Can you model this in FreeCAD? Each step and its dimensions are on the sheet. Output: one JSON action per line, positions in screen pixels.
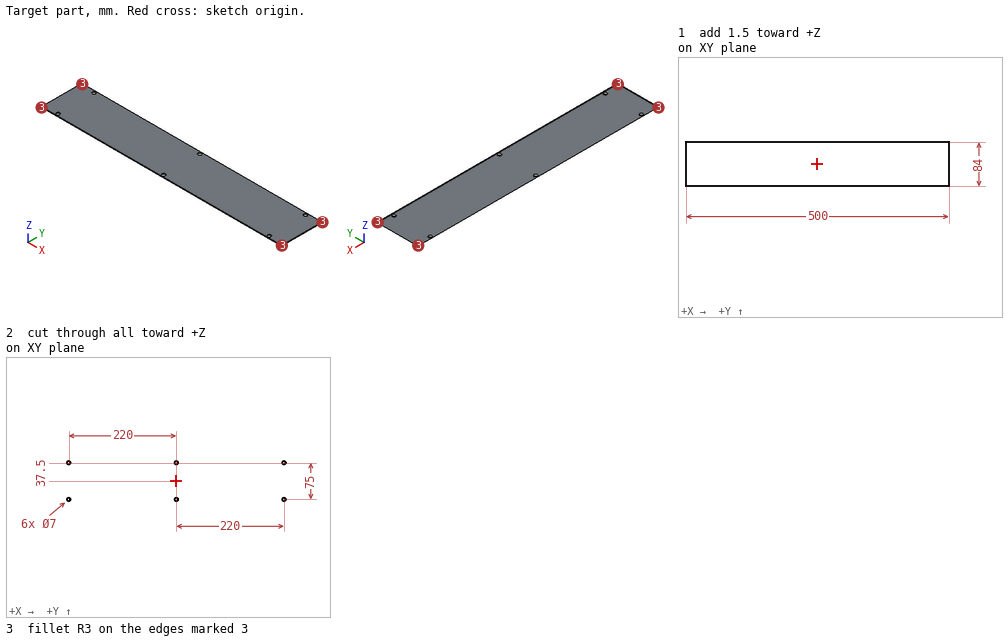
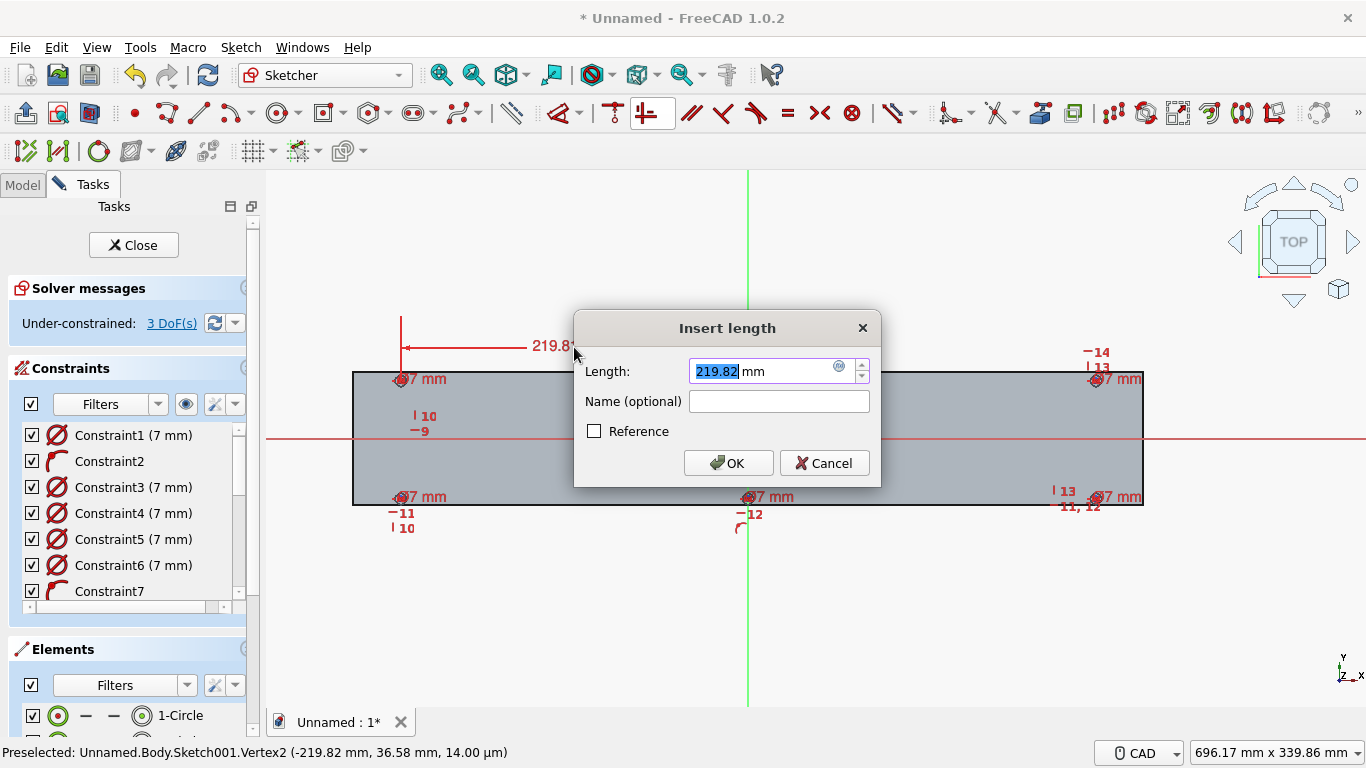
{"action": "type", "text": "220"}
{"action": "key", "text": "Return"}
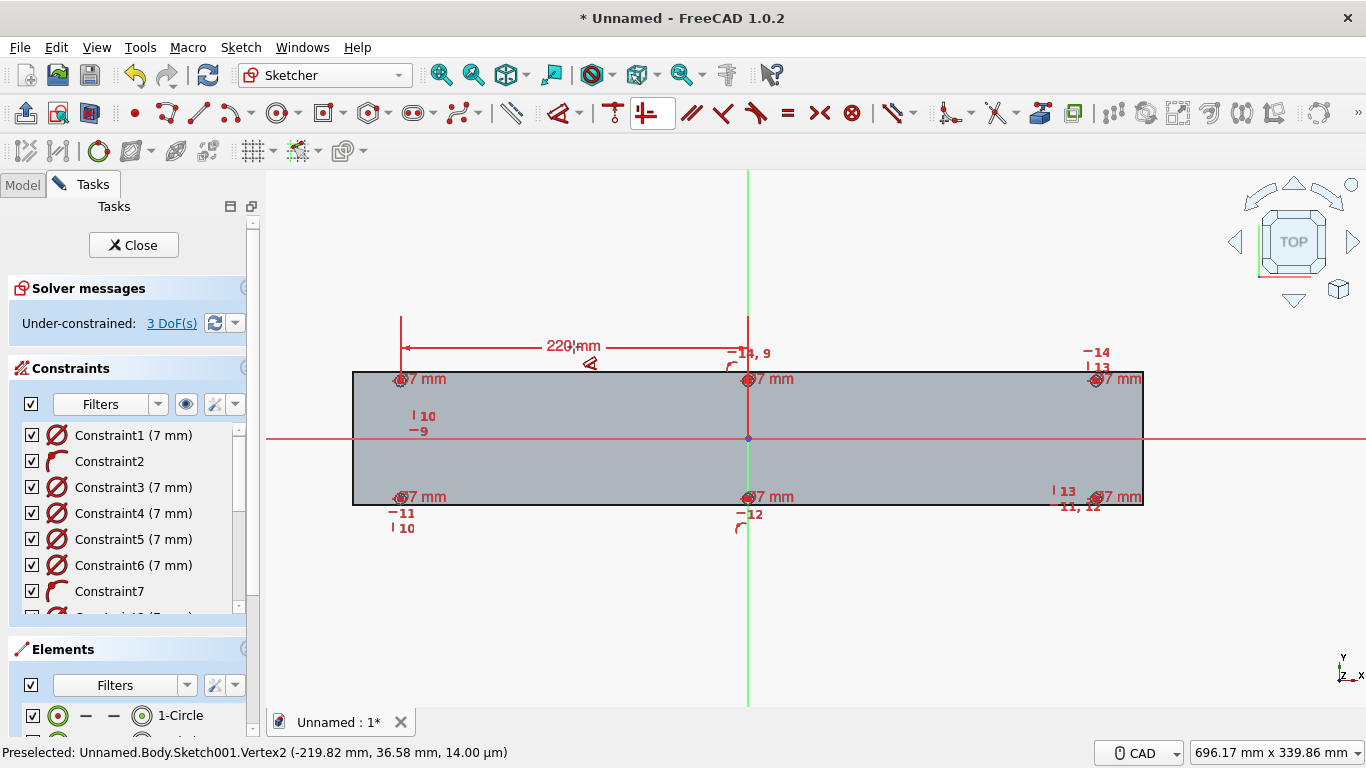
{"action": "left_click", "coordinate": [1096, 499]}
{"action": "left_click", "coordinate": [922, 533]}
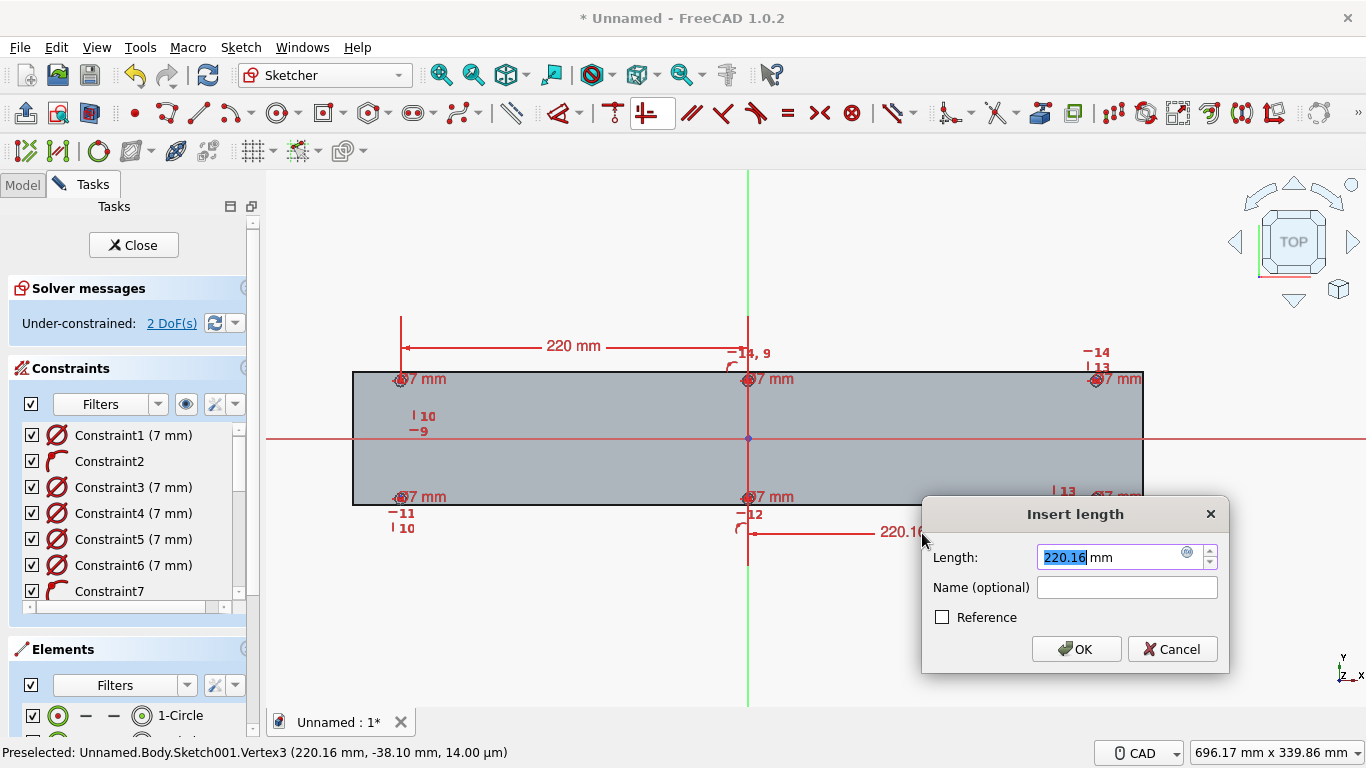
{"action": "type", "text": "220"}
{"action": "key", "text": "Return"}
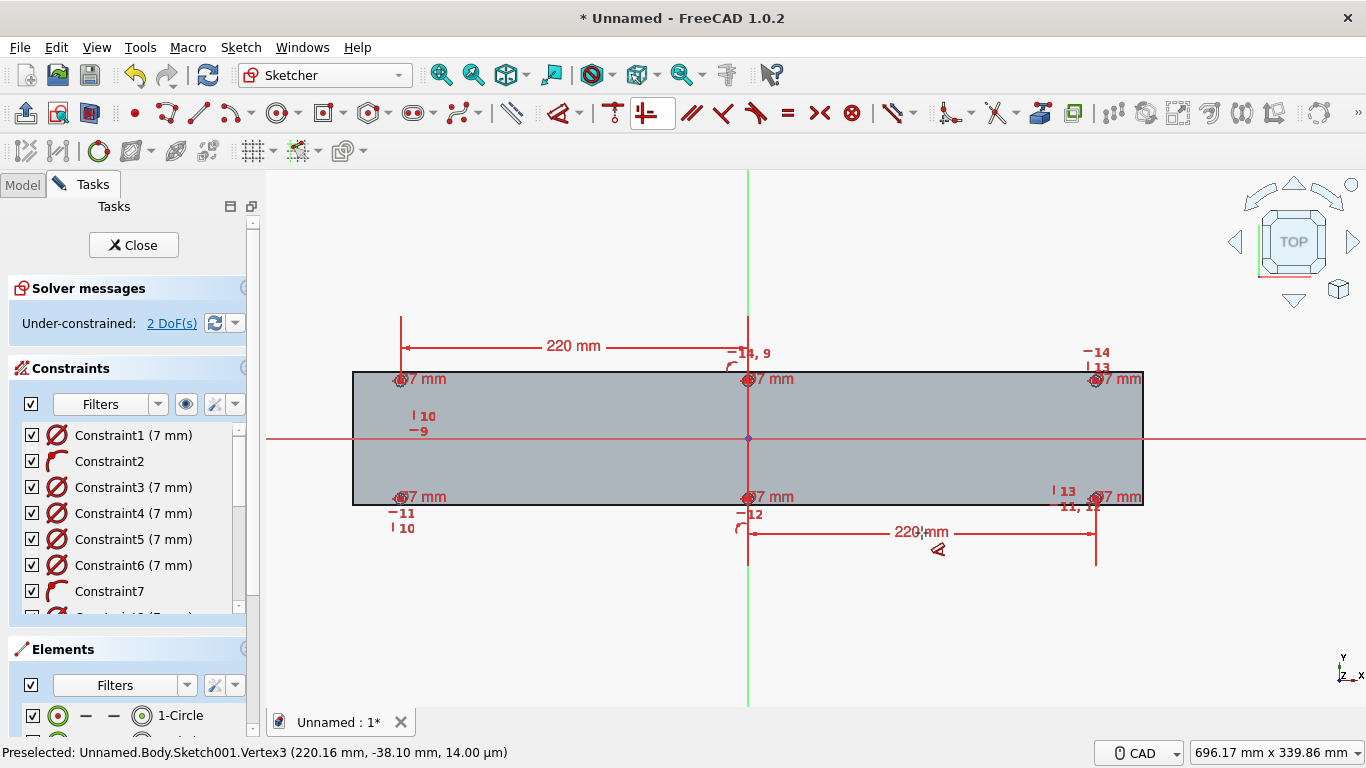
{"action": "left_click", "coordinate": [748, 381]}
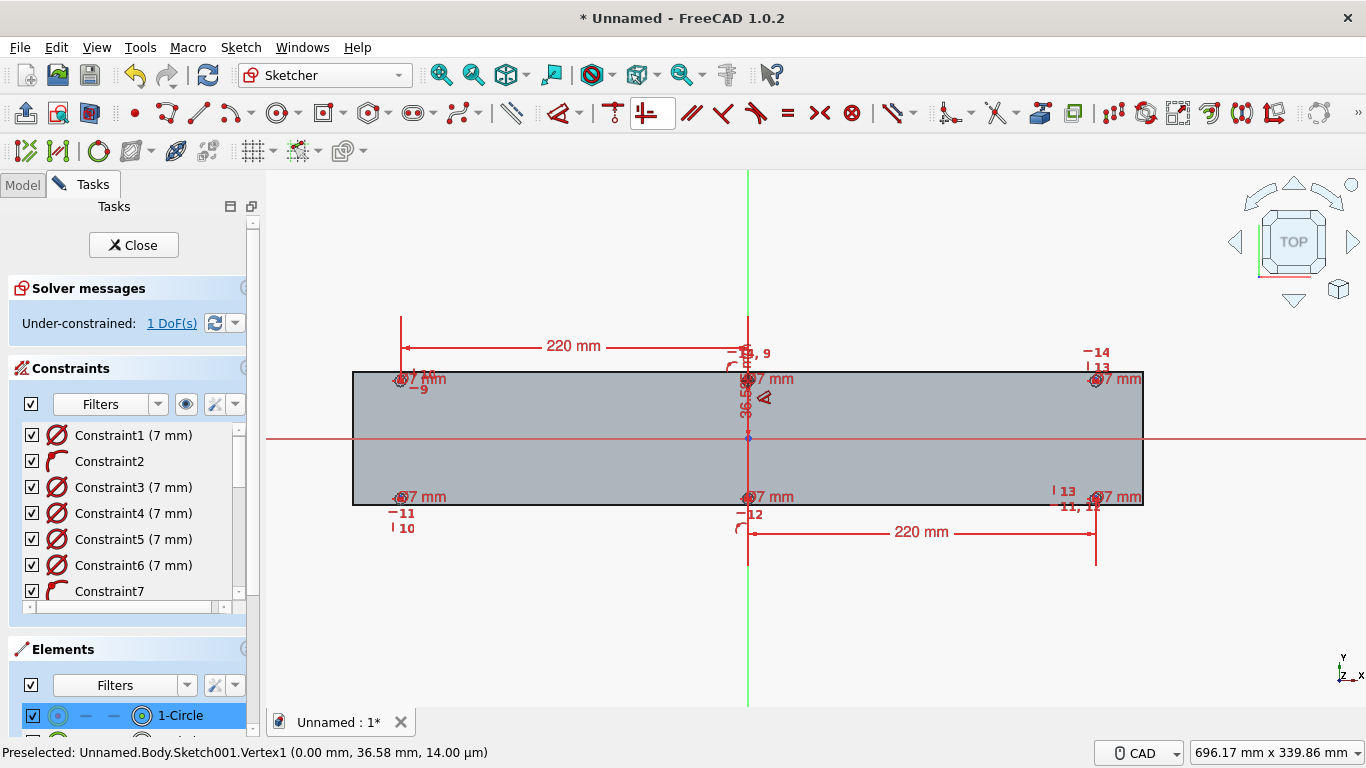
{"action": "left_click", "coordinate": [1096, 499]}
{"action": "left_click", "coordinate": [1130, 413]}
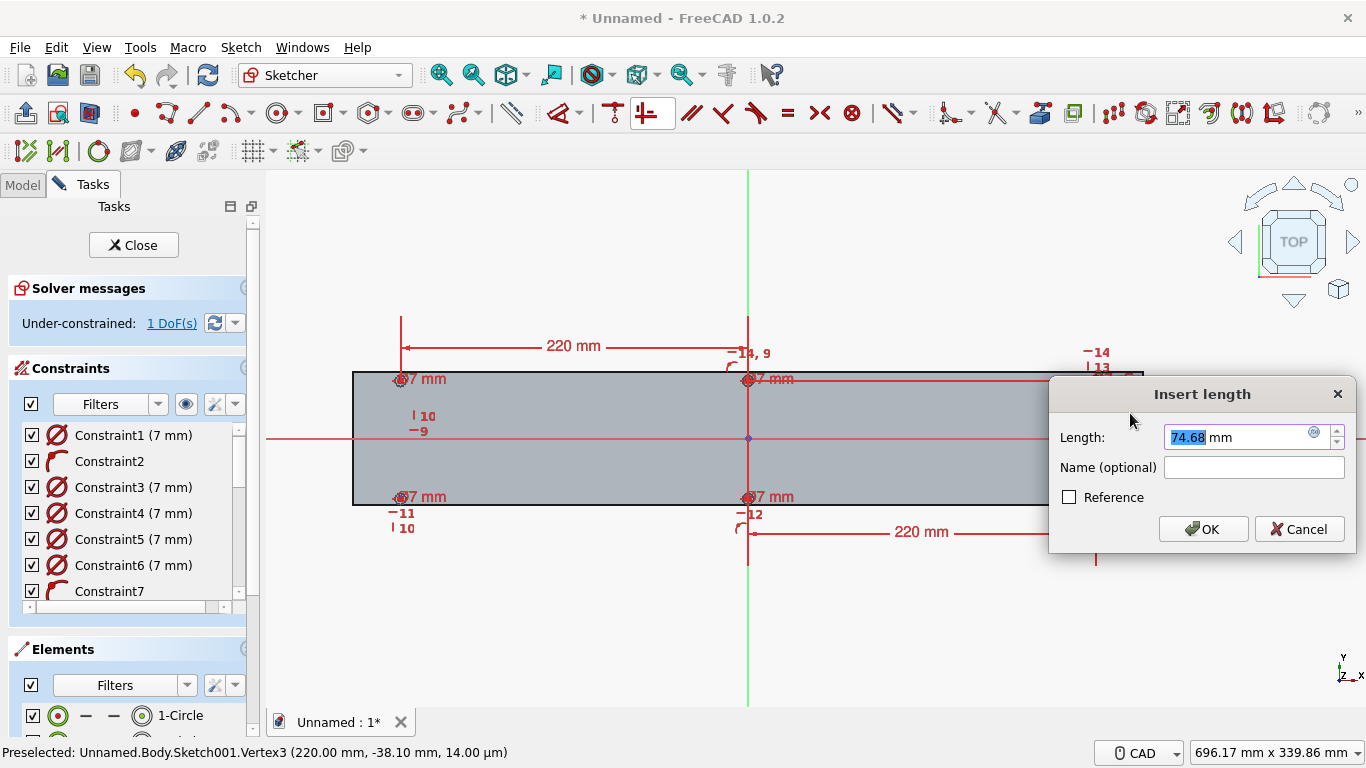
{"action": "type", "text": "75"}
{"action": "key", "text": "Return"}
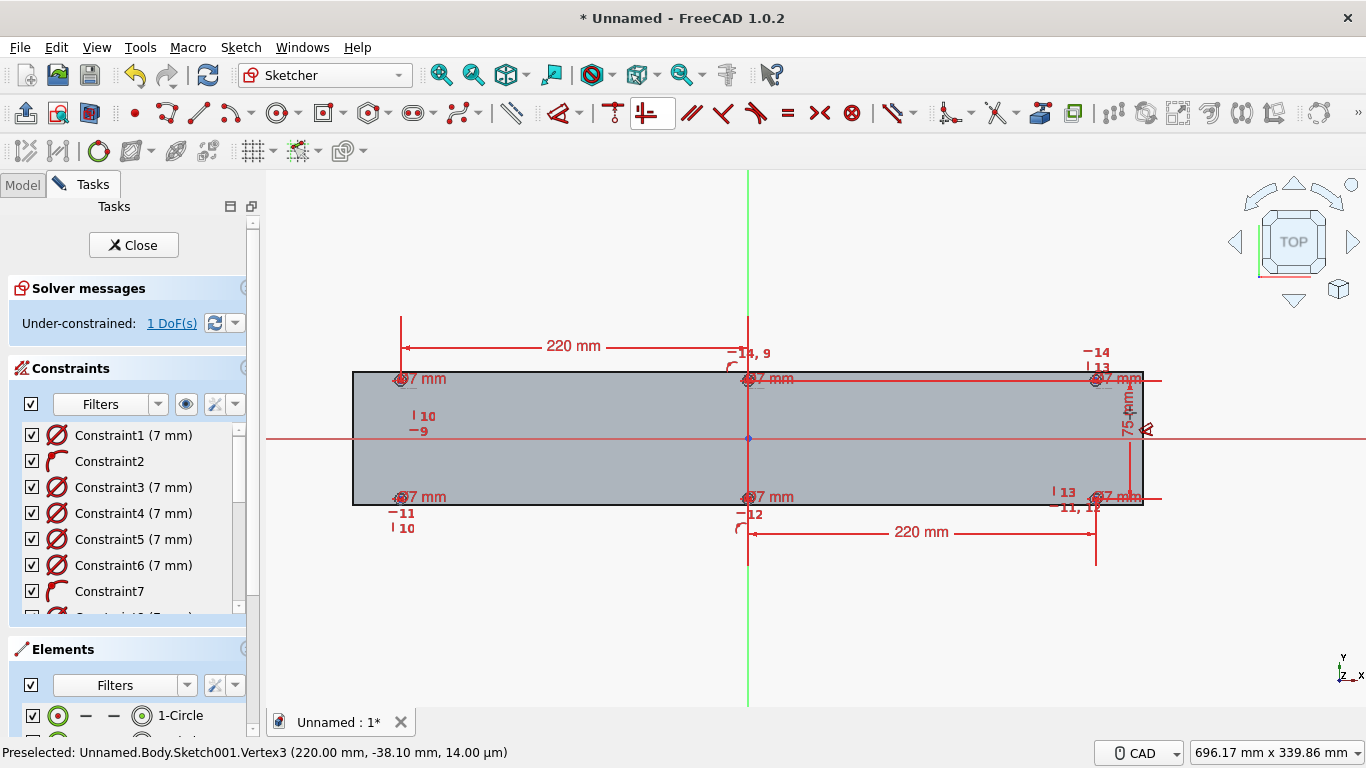
{"action": "left_click", "coordinate": [748, 381]}
{"action": "left_click", "coordinate": [782, 410]}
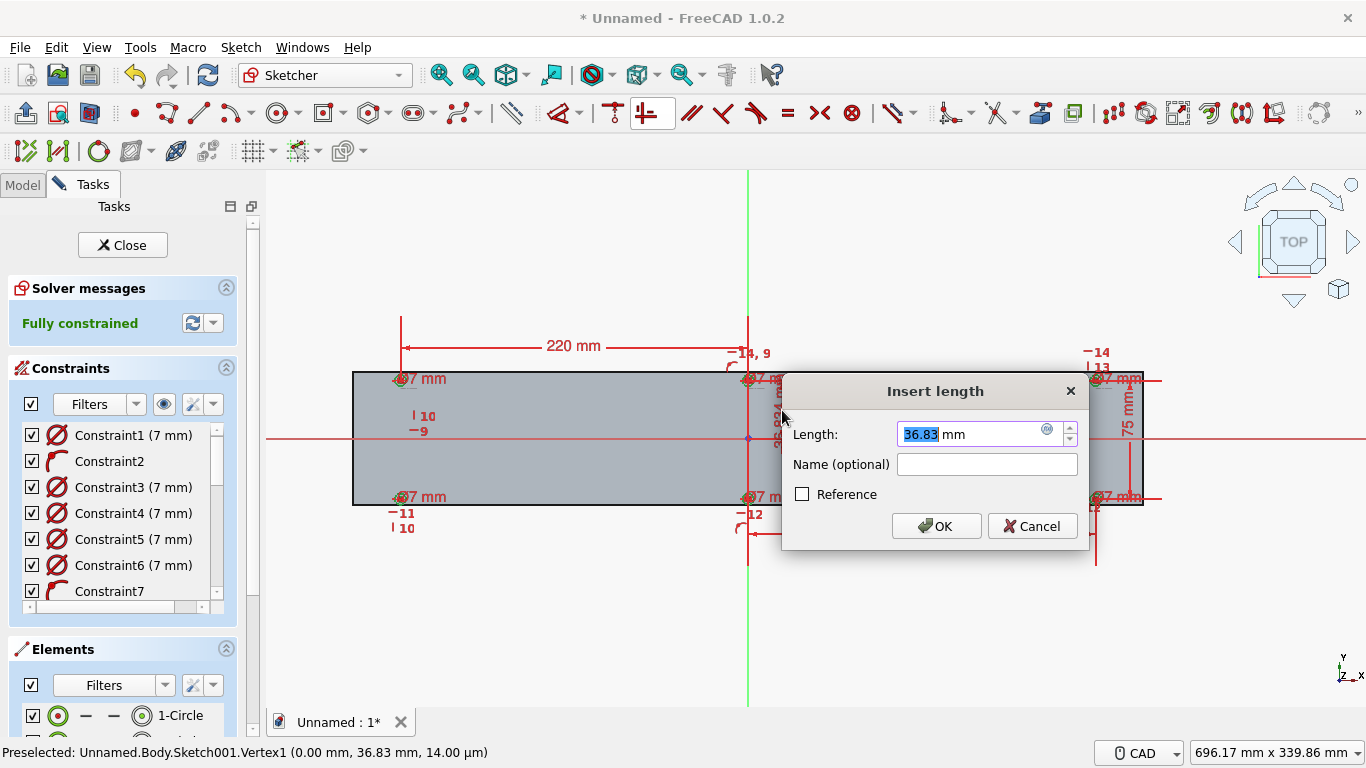
{"action": "type", "text": "37.5"}
{"action": "key", "text": "Return"}
{"action": "key", "text": "Escape"}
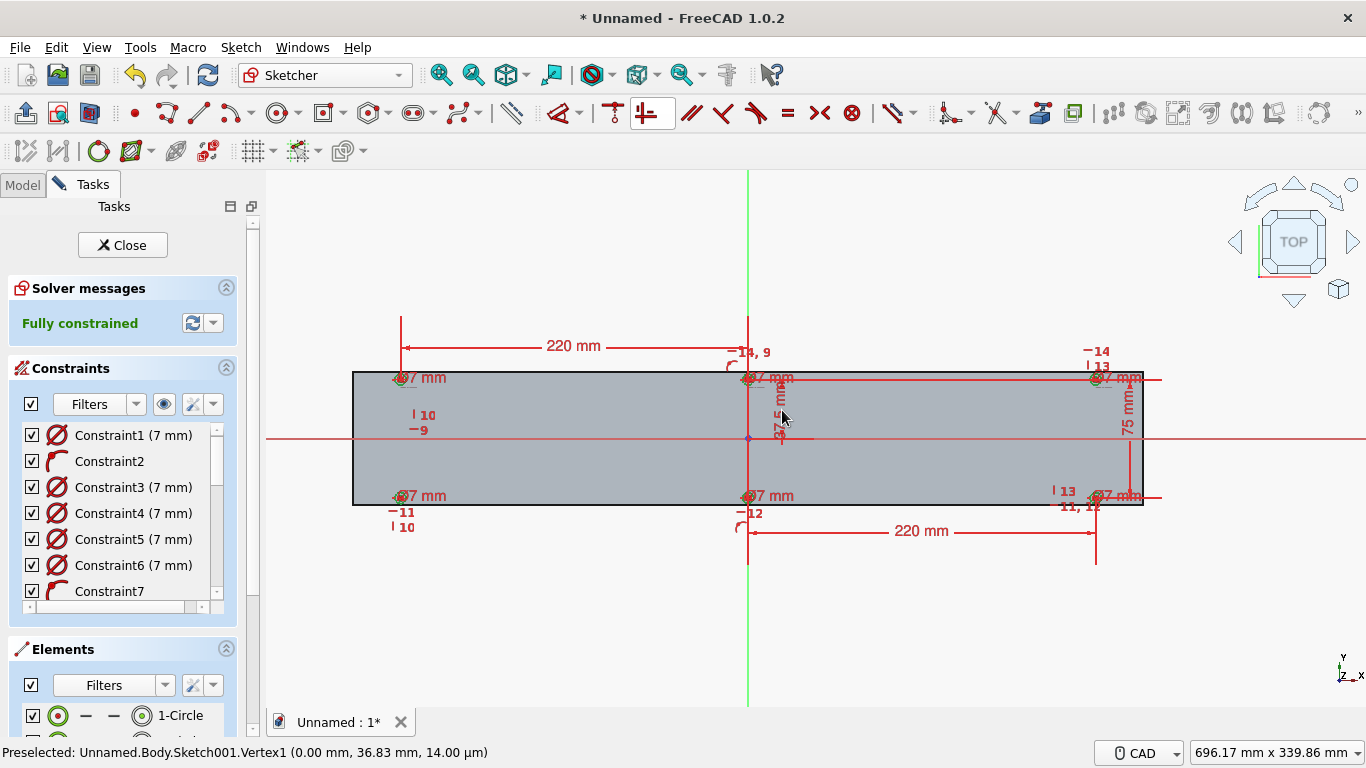
{"action": "left_click", "coordinate": [123, 245]}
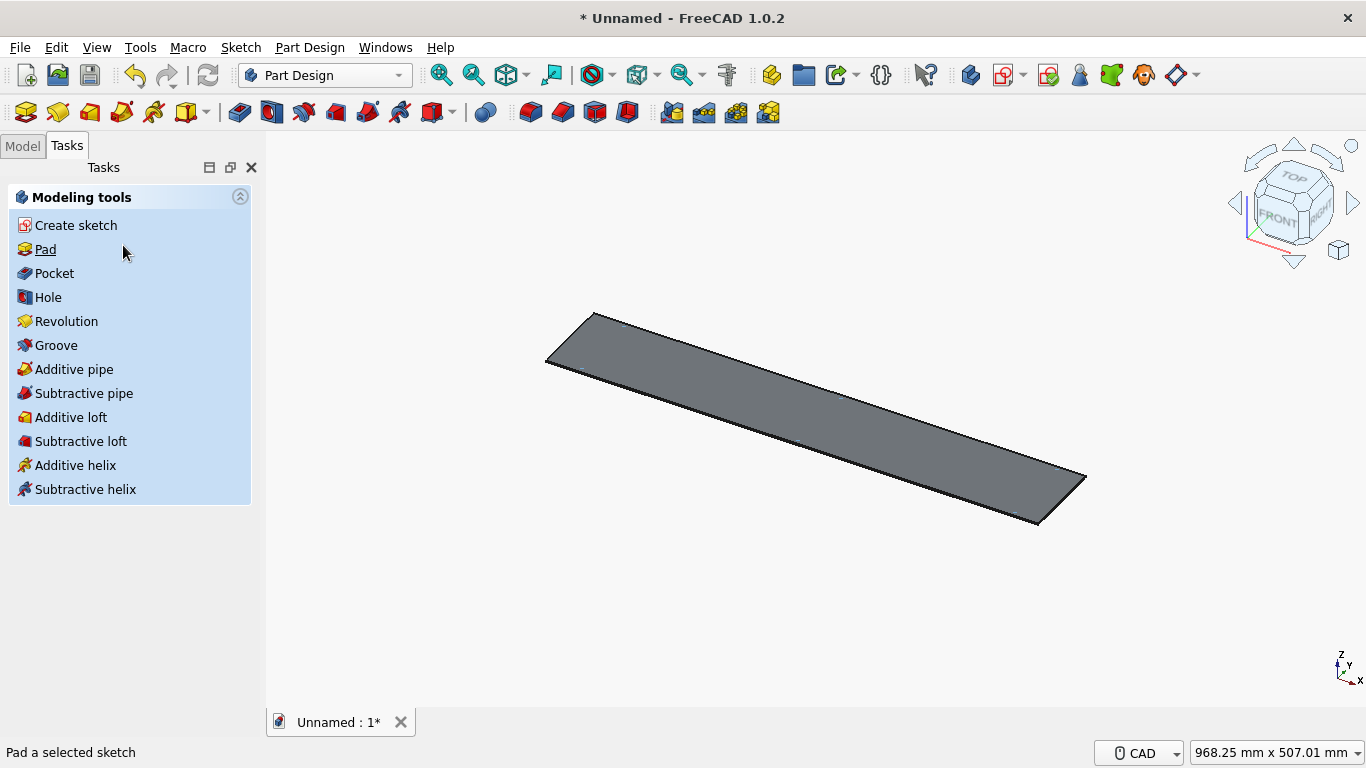
{"action": "left_click", "coordinate": [240, 112]}